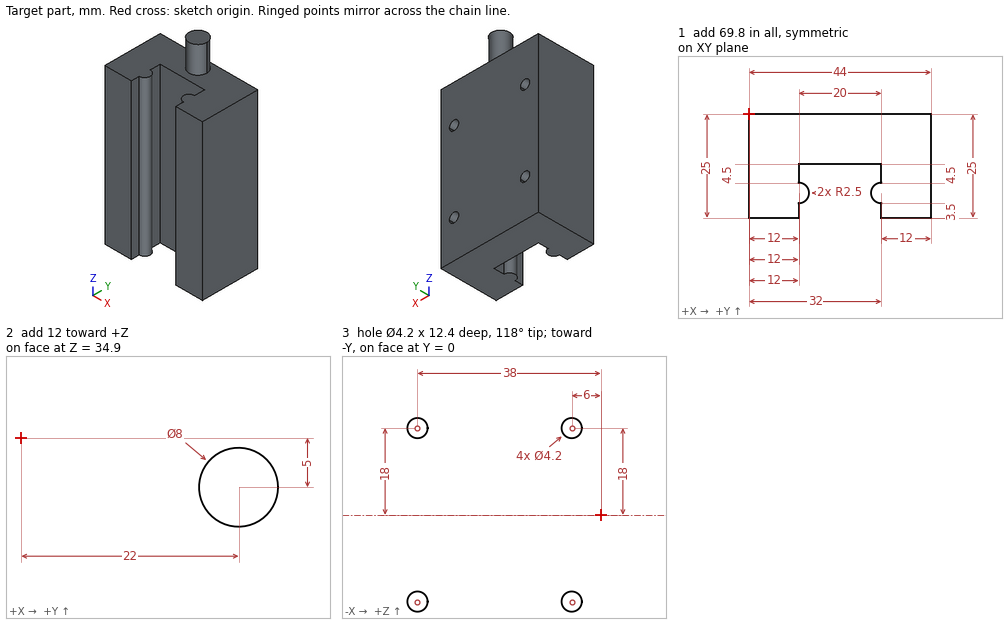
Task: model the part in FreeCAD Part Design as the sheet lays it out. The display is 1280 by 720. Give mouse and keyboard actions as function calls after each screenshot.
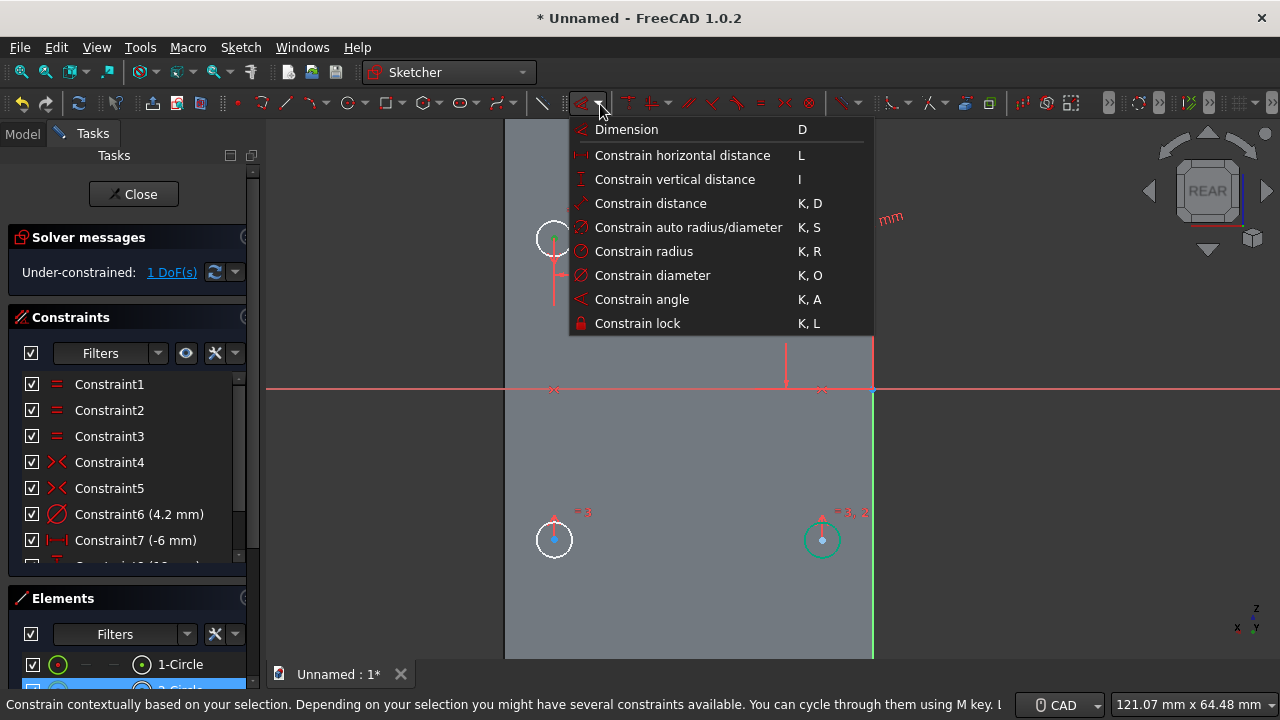
click(722, 179)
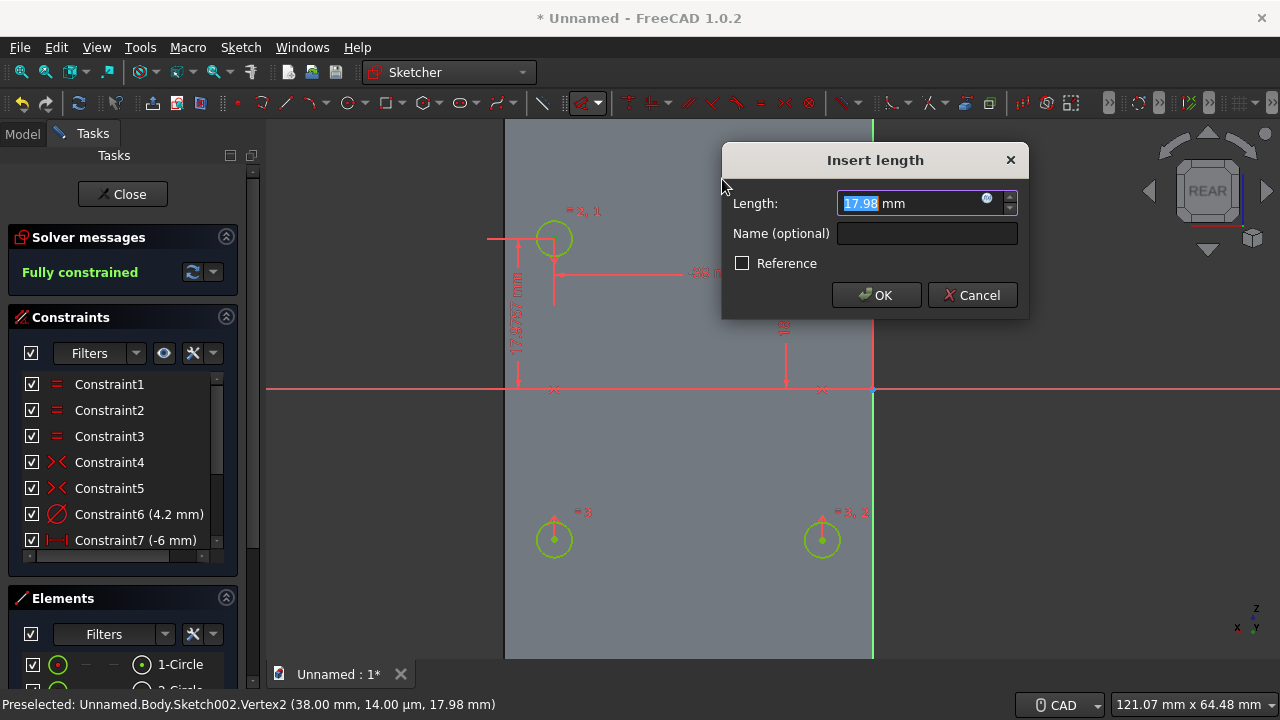
text(18)
key(Return)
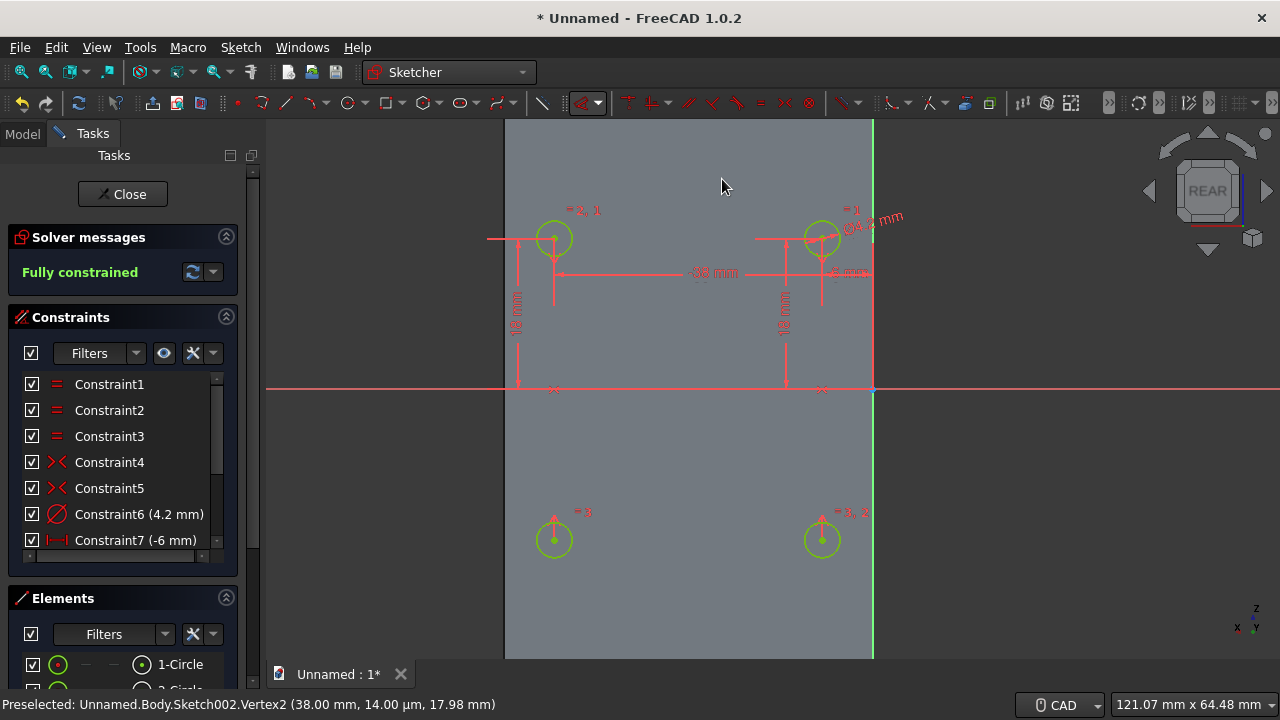
click(123, 194)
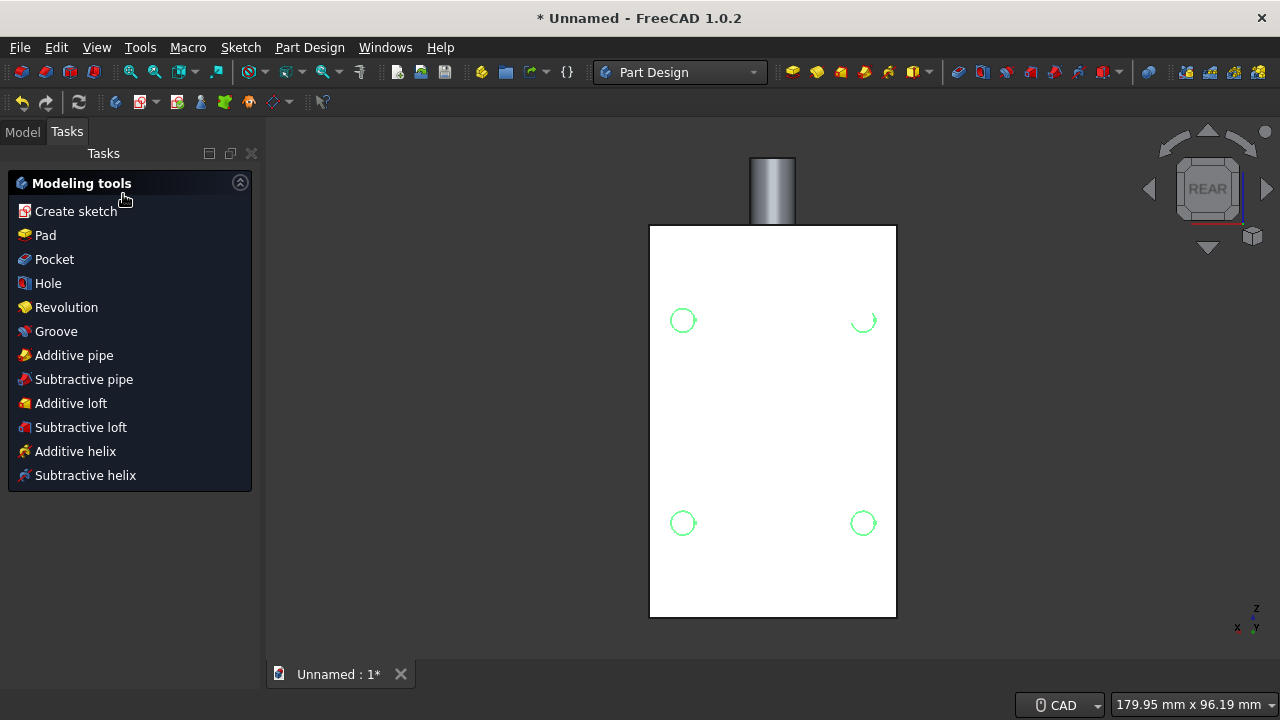
click(984, 72)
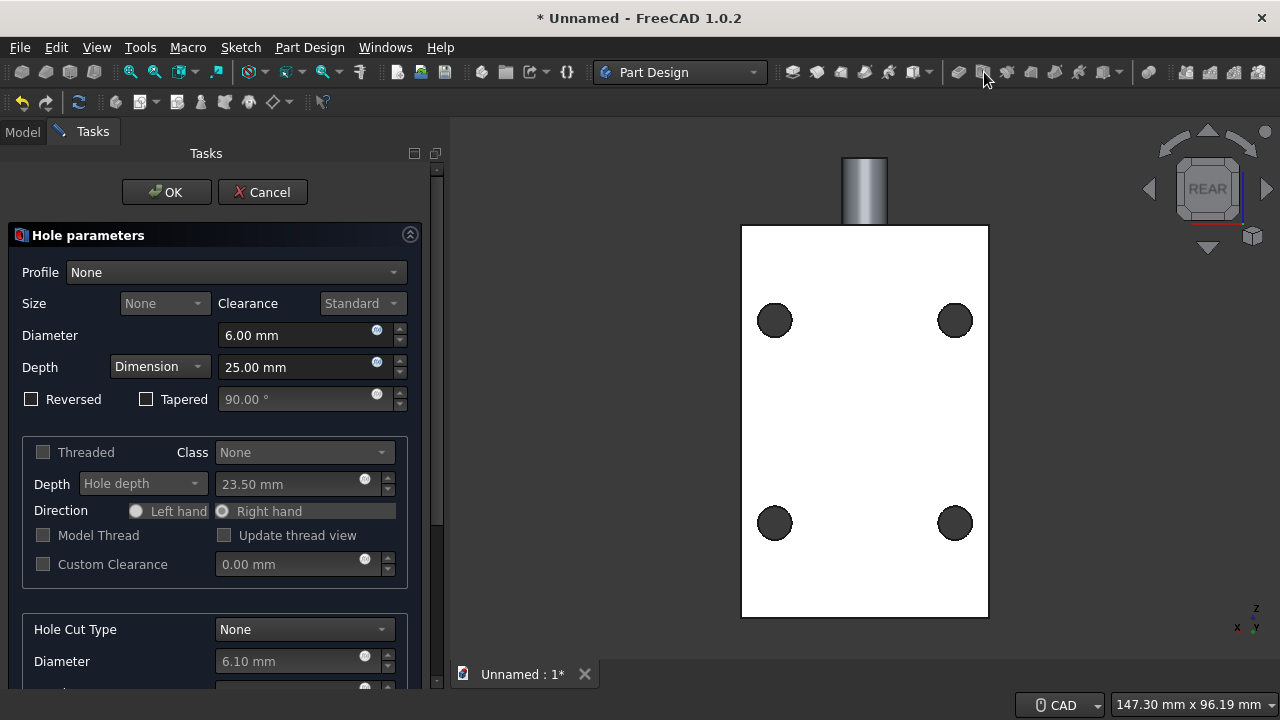
triple_click(305, 335)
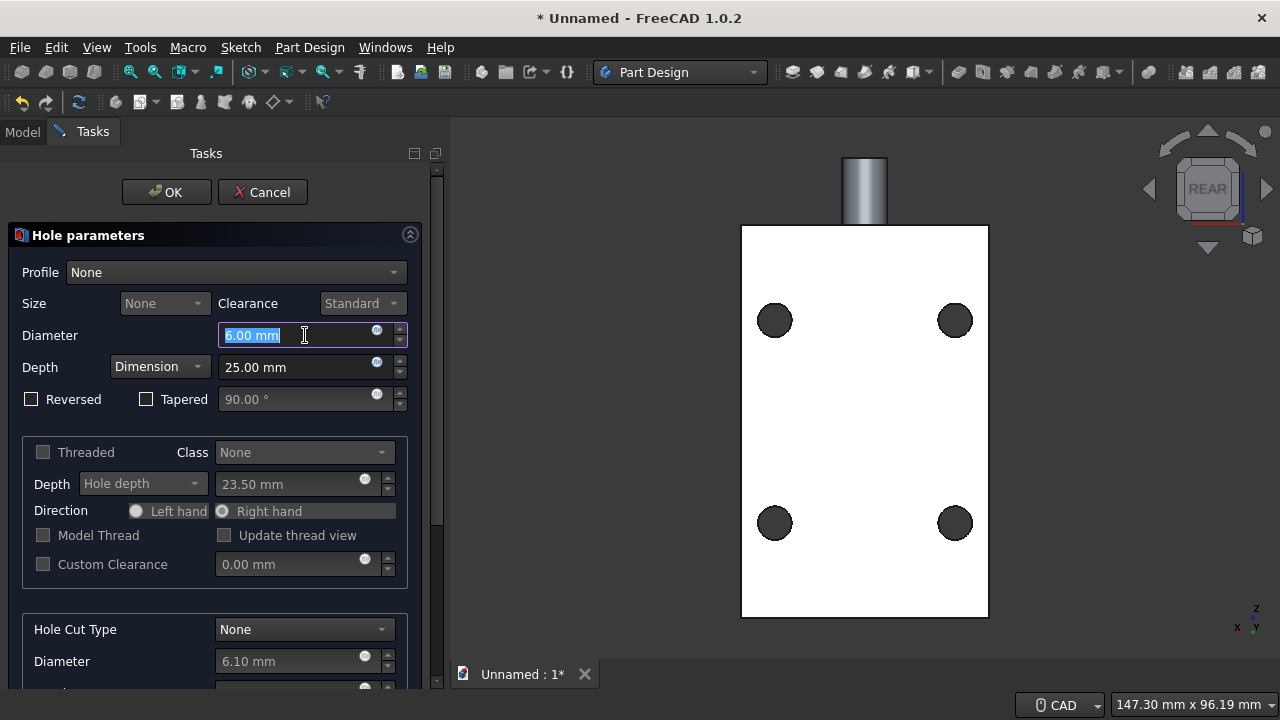
text(4.2)
key(Tab)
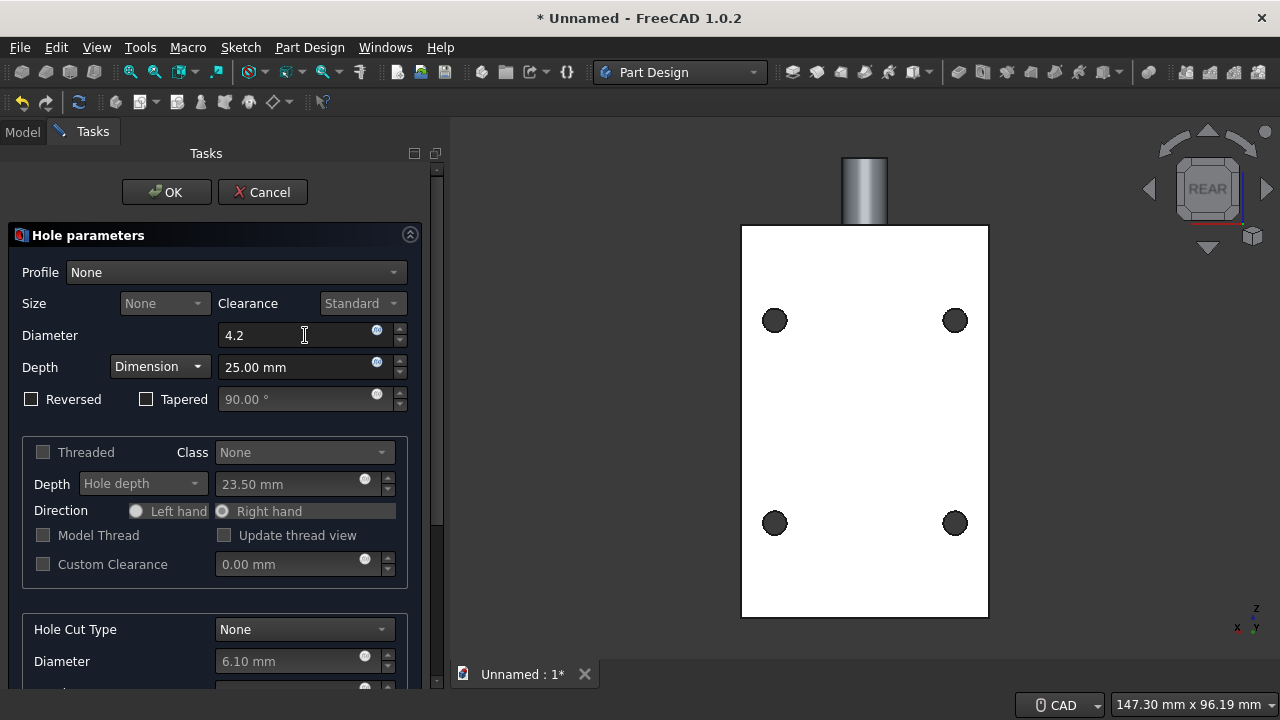
triple_click(305, 367)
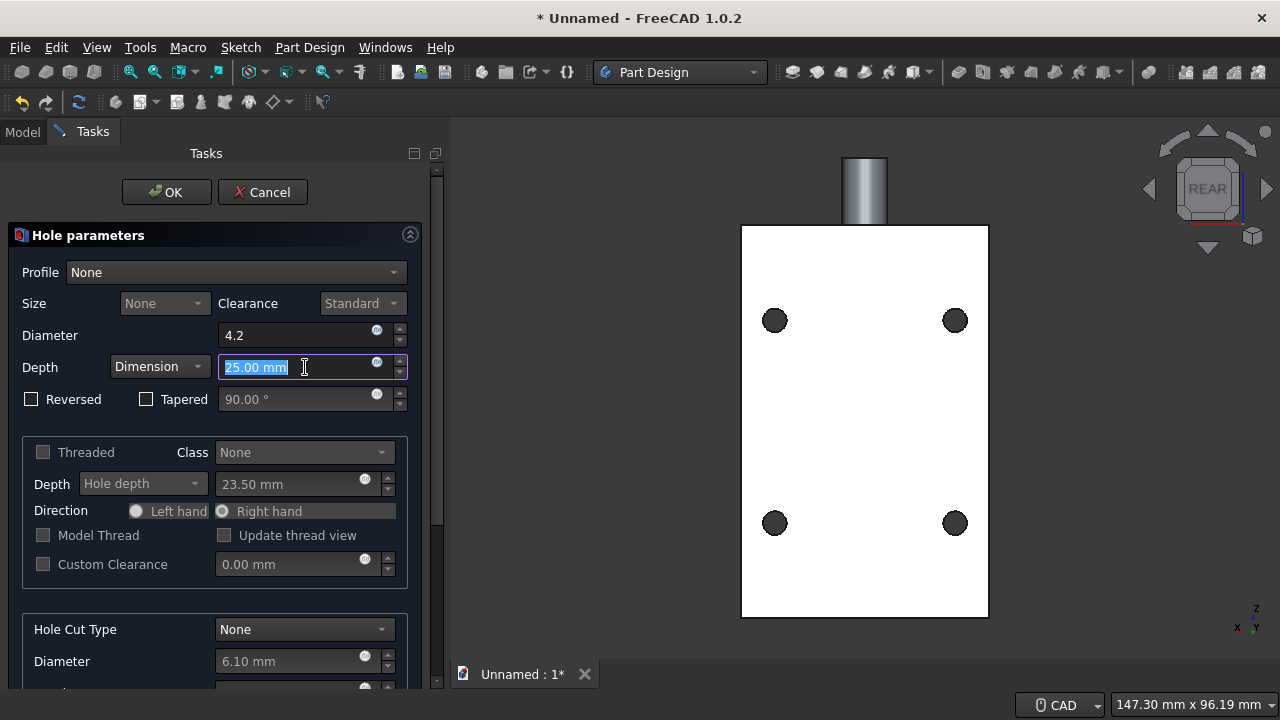
text(12.4)
key(Tab)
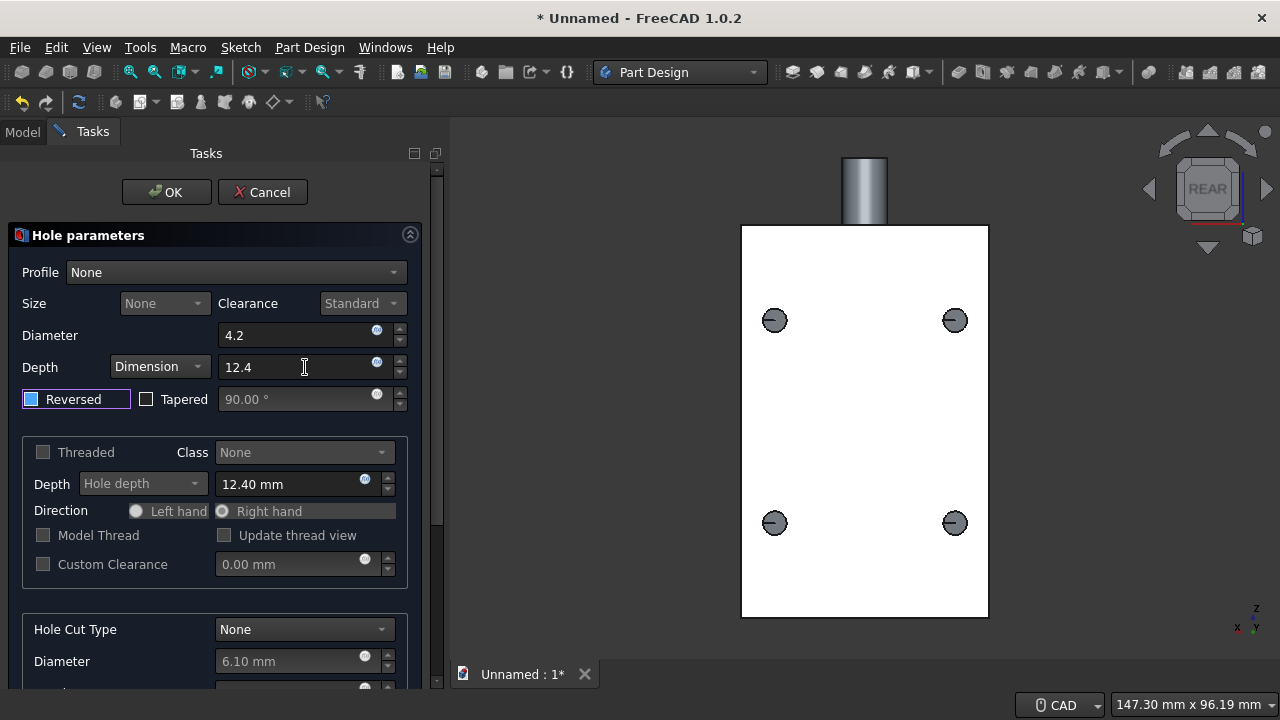
click(167, 192)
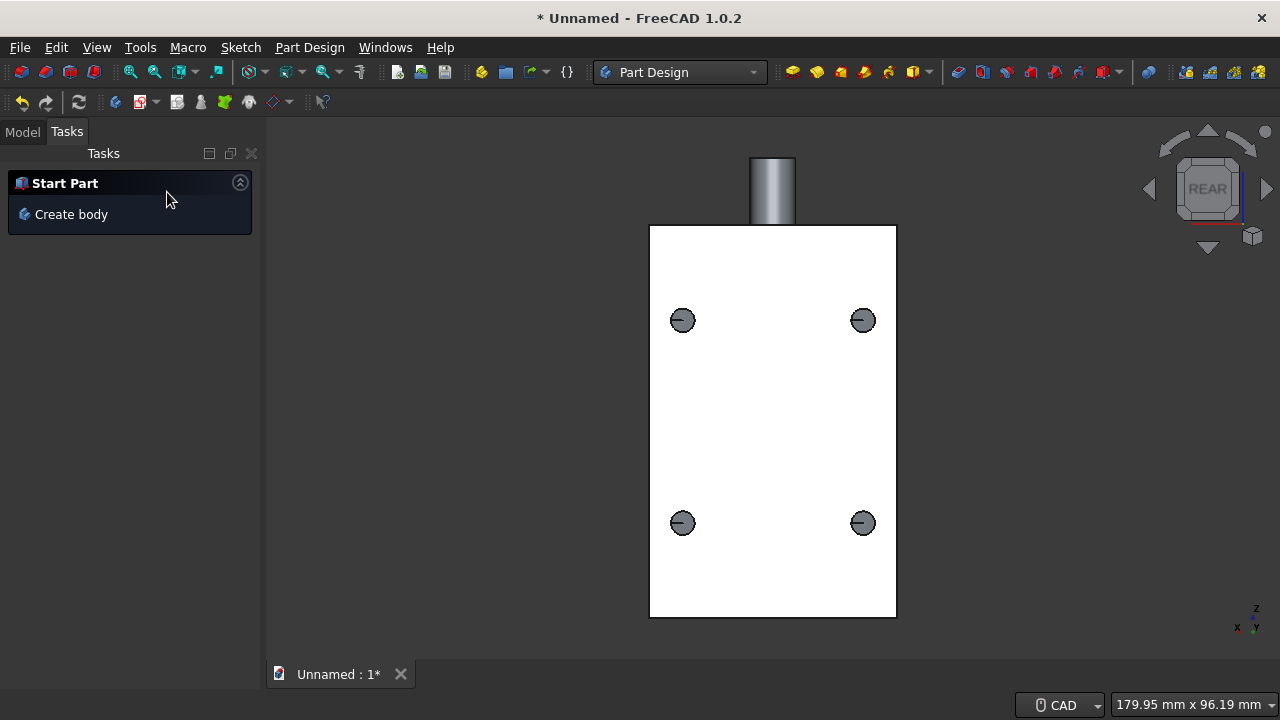
key(0)